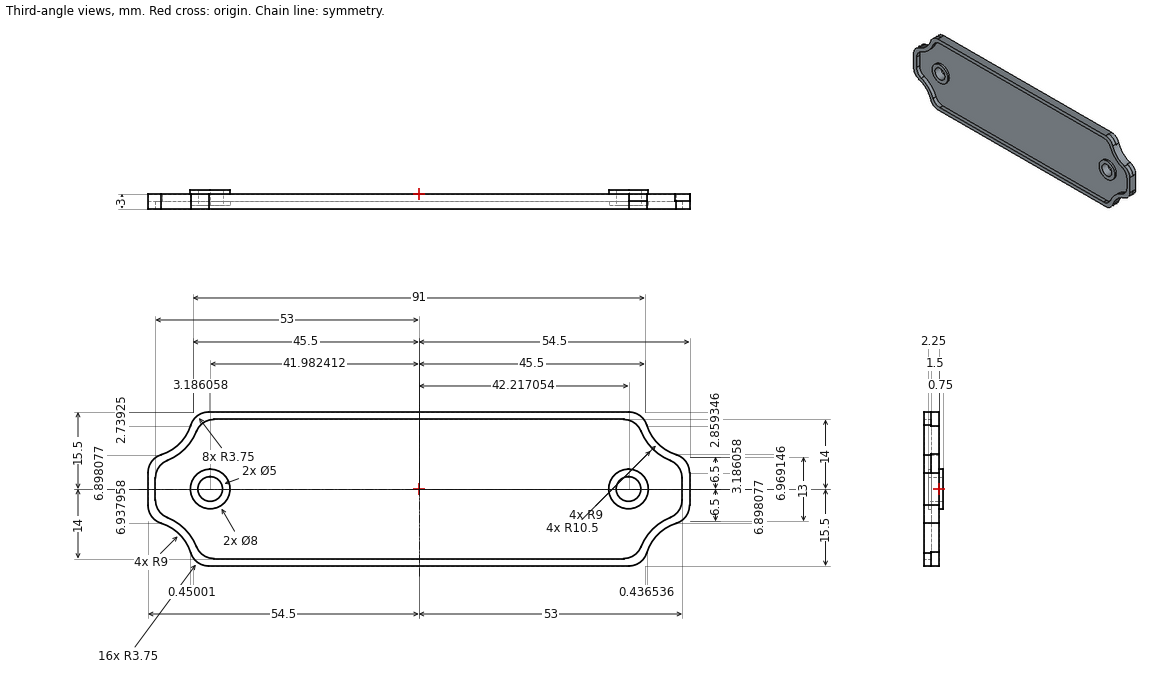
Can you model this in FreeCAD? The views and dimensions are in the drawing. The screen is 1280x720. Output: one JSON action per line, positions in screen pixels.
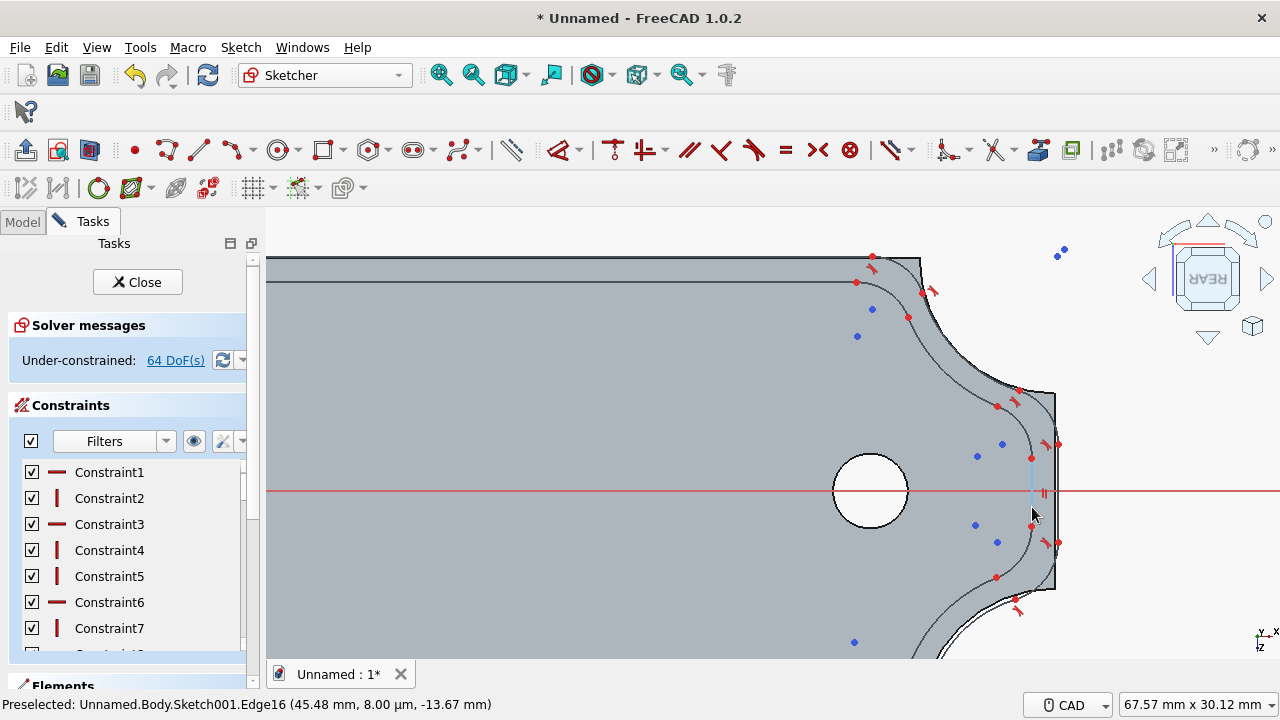
{"action": "left_click", "coordinate": [1032, 506]}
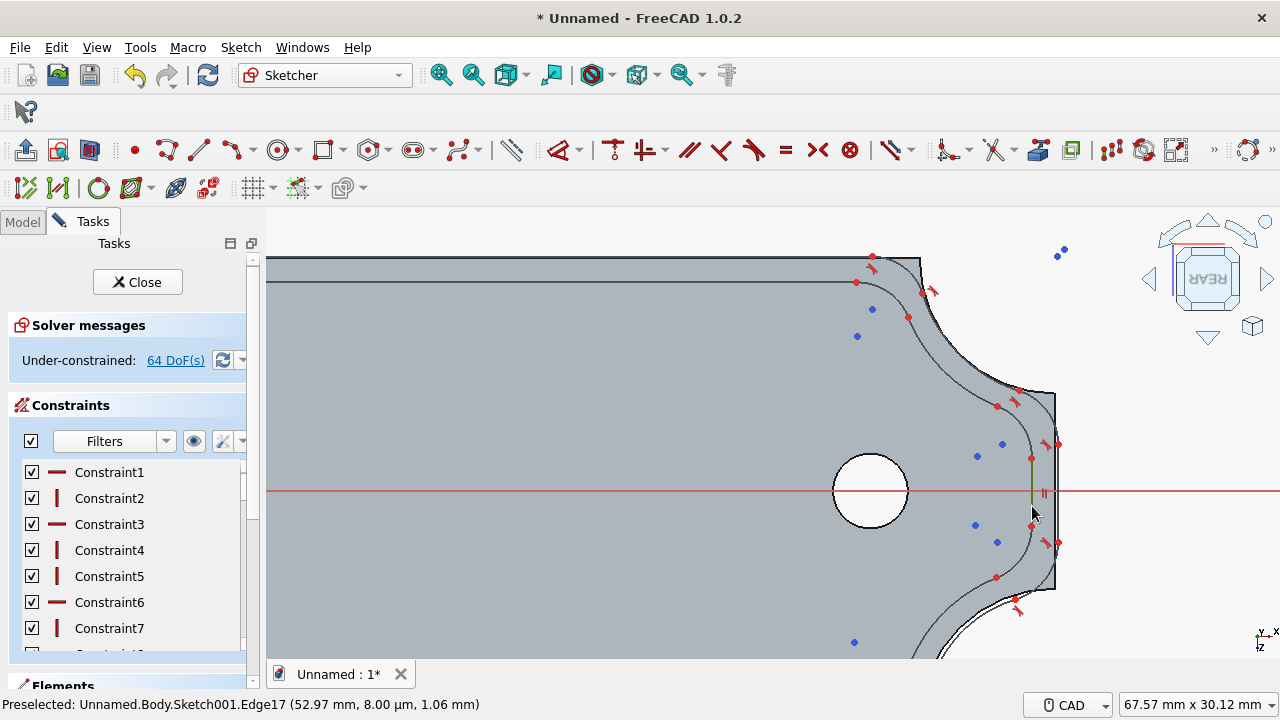
{"action": "left_click", "coordinate": [1013, 567]}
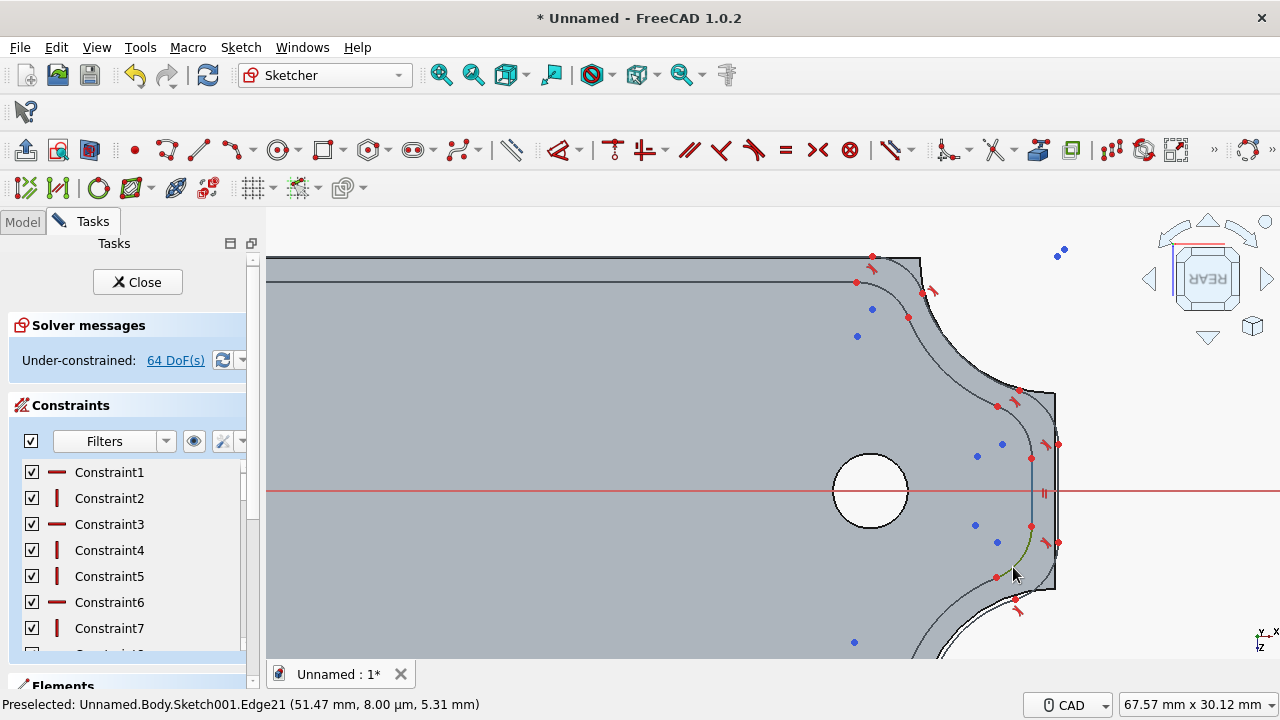
{"action": "left_click", "coordinate": [754, 150]}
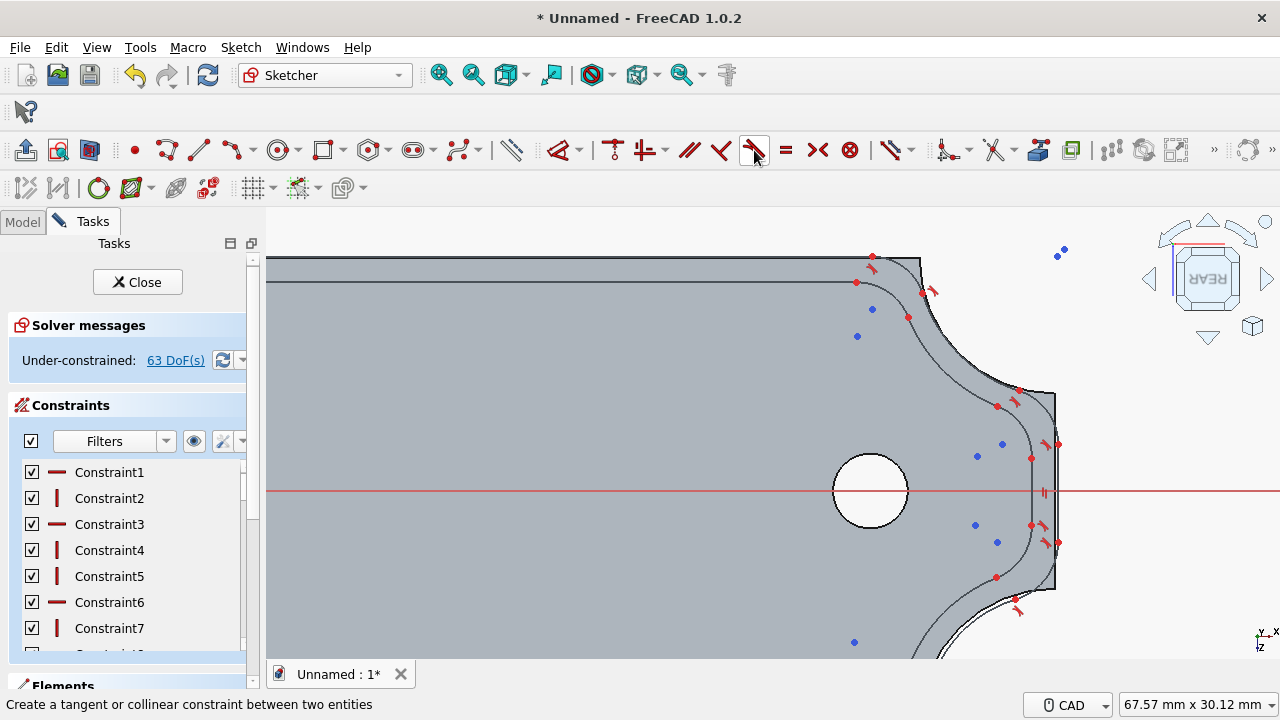
{"action": "left_click", "coordinate": [1032, 478]}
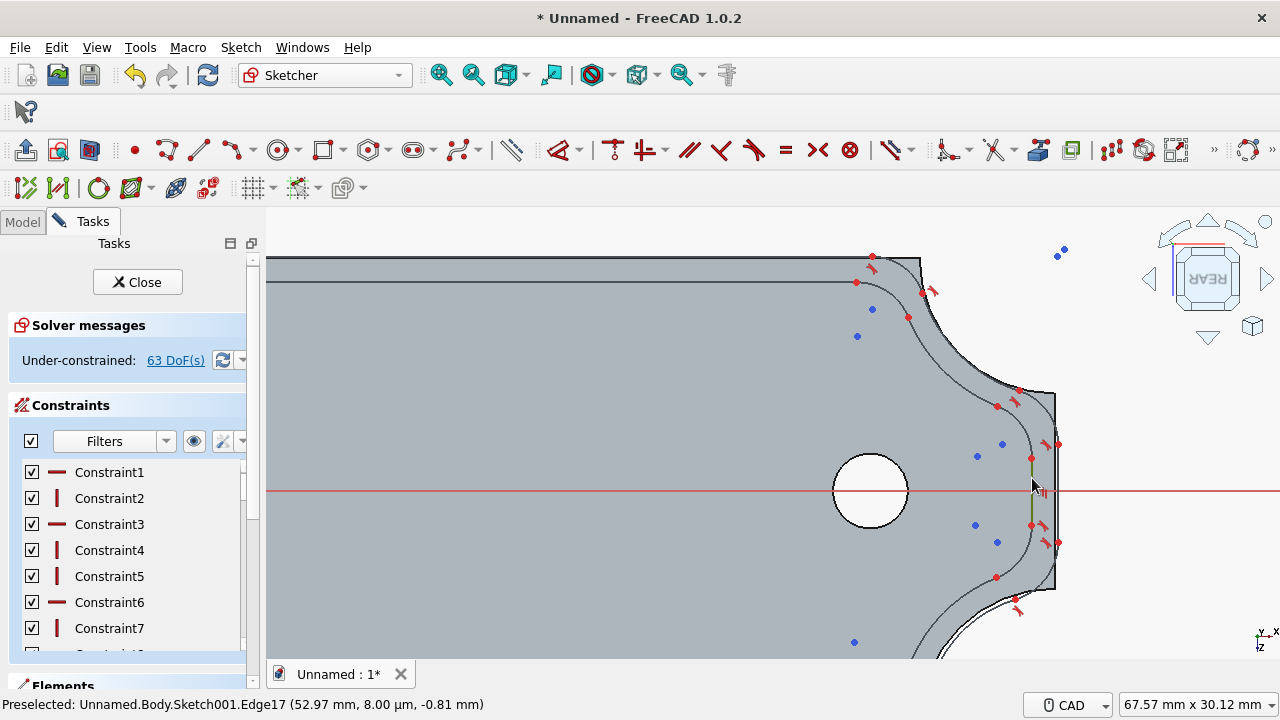
{"action": "left_click", "coordinate": [1029, 439]}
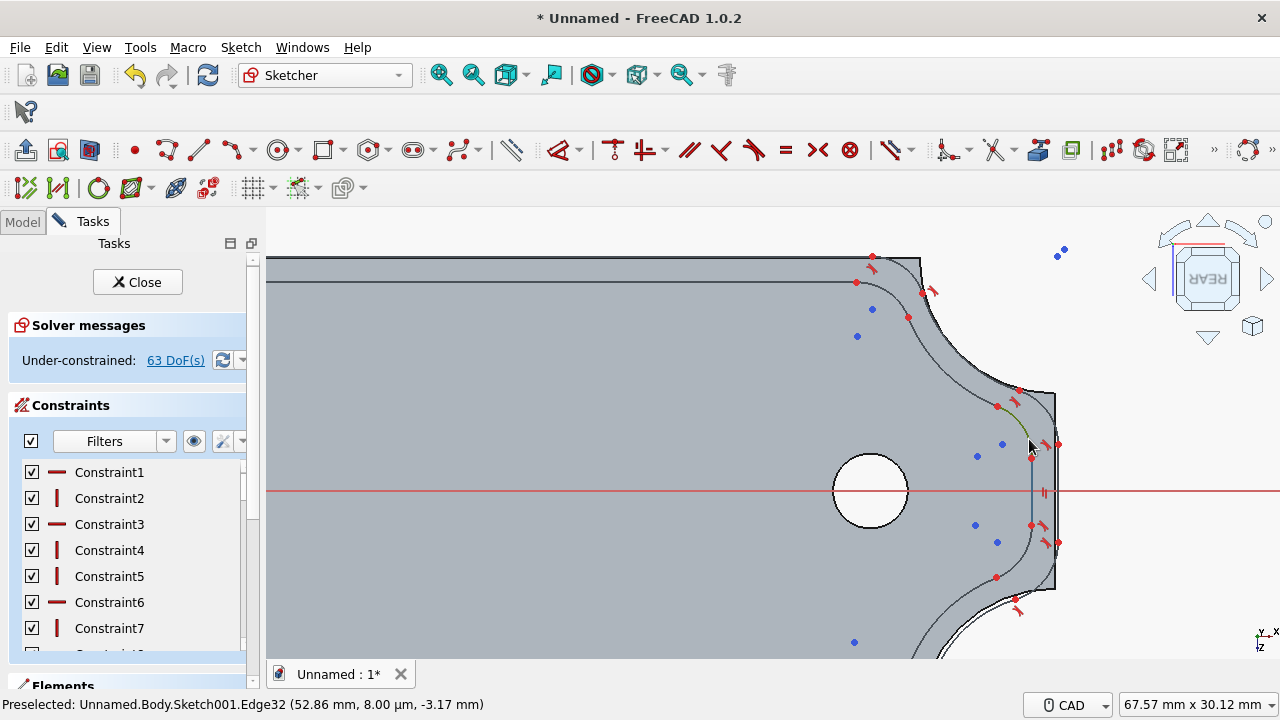
{"action": "left_click", "coordinate": [754, 150]}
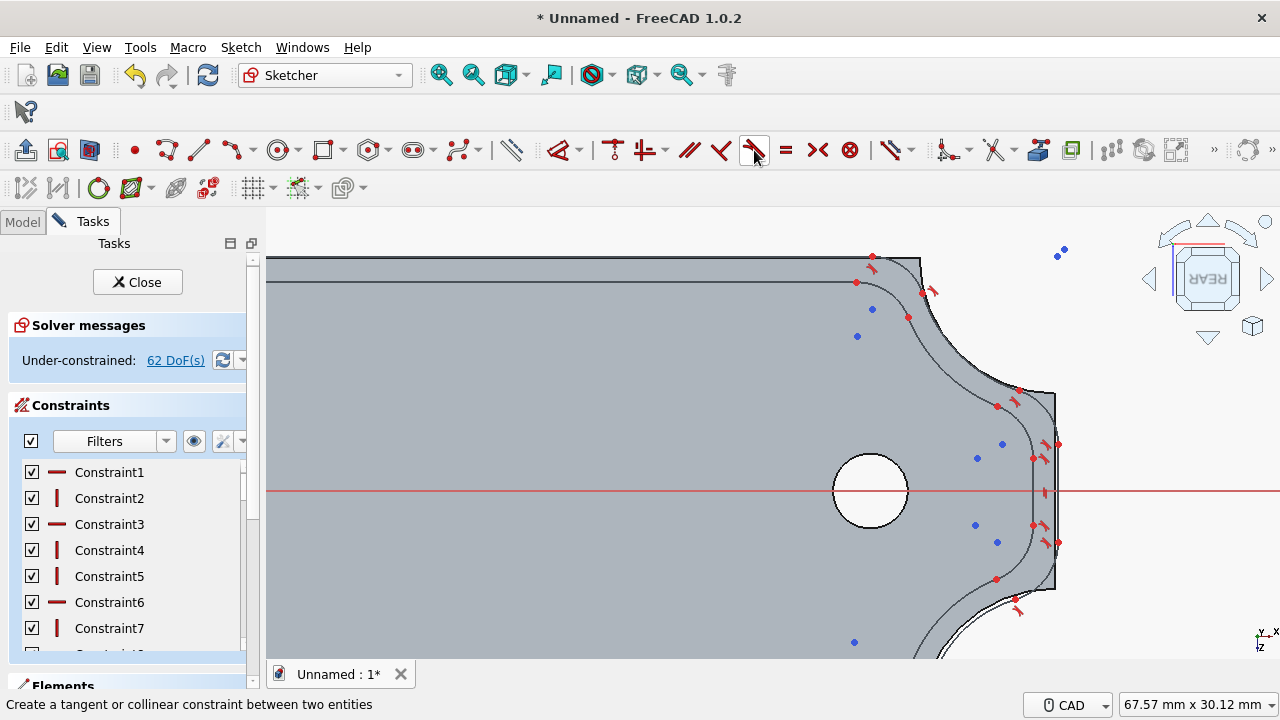
{"action": "scroll", "coordinate": [977, 399], "scroll_direction": "down", "scroll_amount": 5}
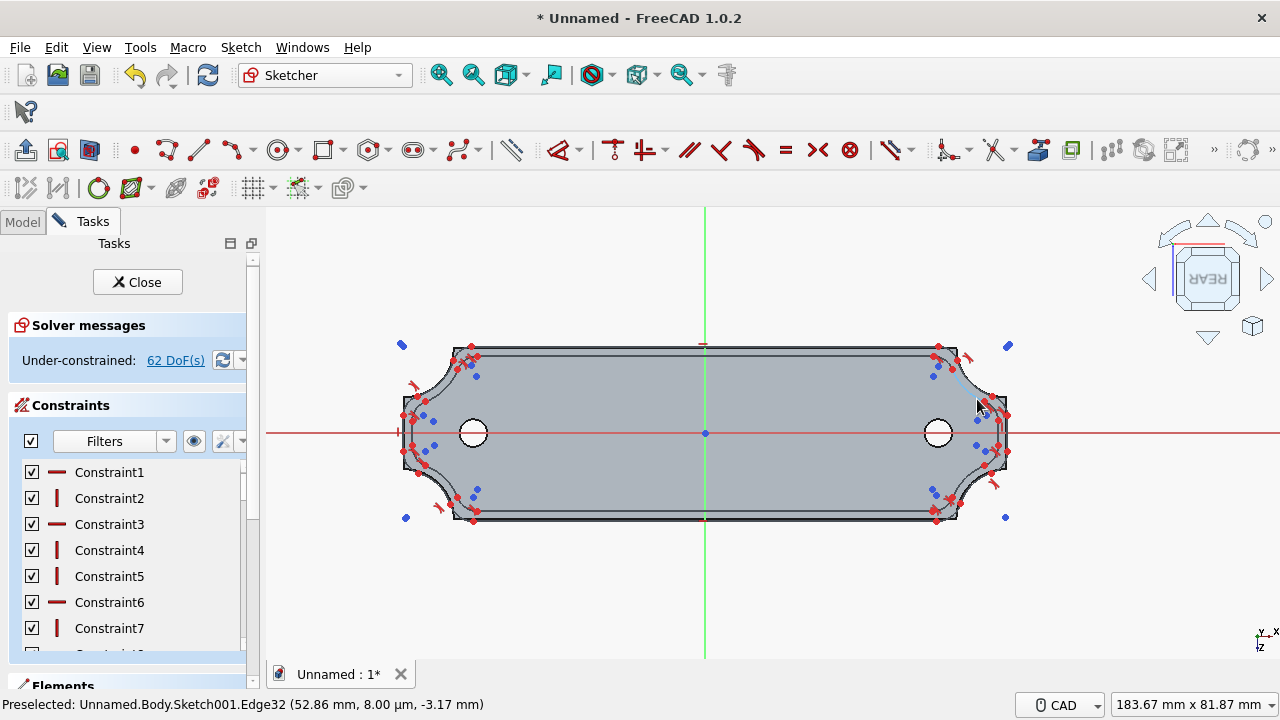
{"action": "scroll", "coordinate": [796, 511], "scroll_direction": "up", "scroll_amount": 2}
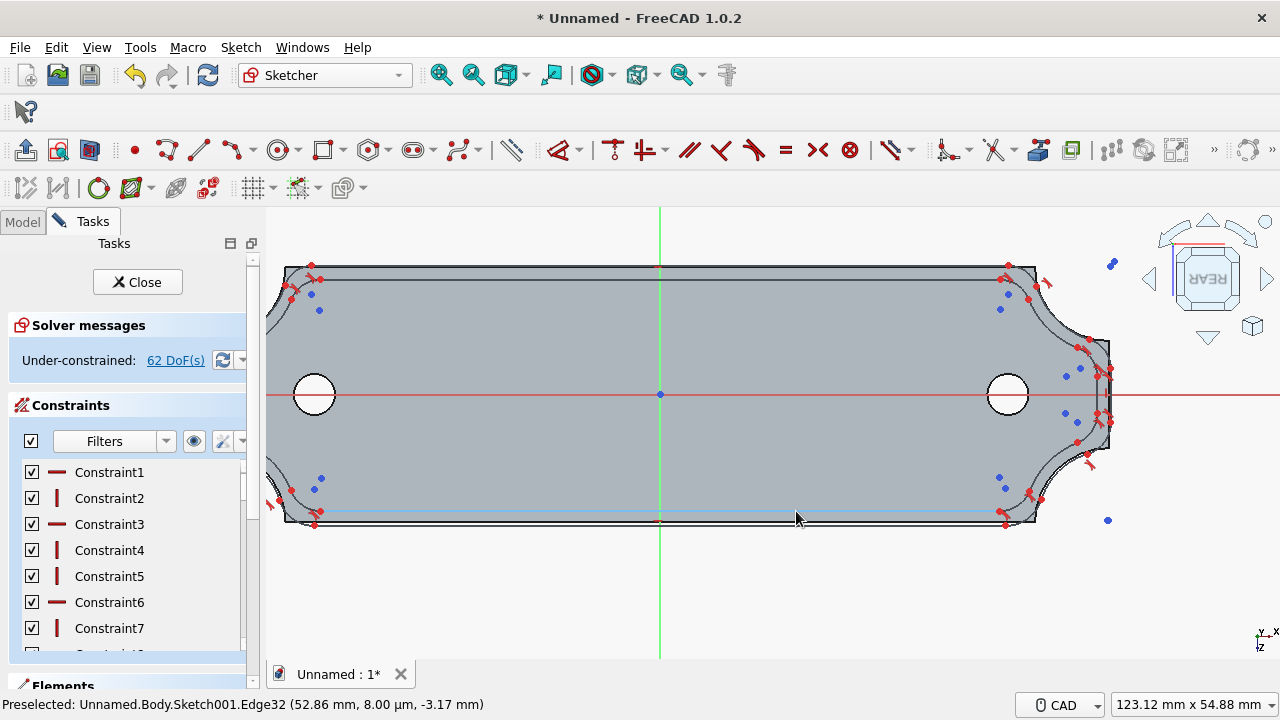
{"action": "left_click", "coordinate": [796, 511]}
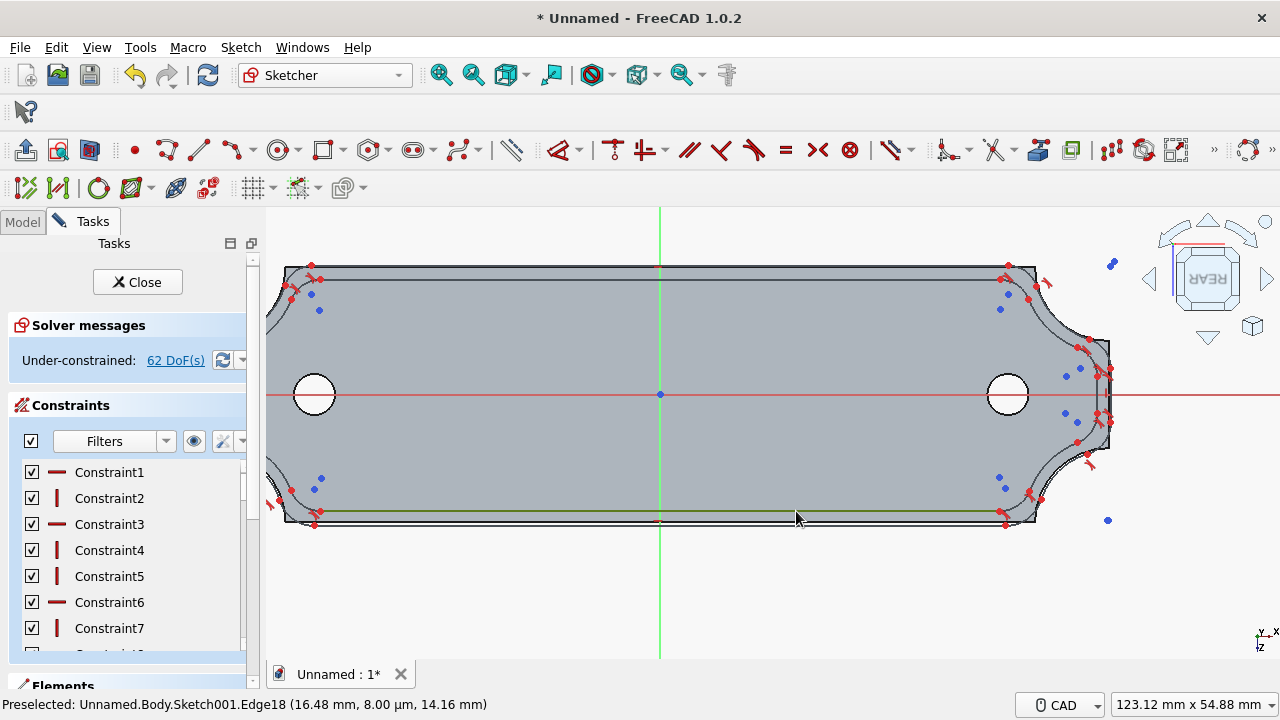
{"action": "left_click", "coordinate": [1024, 501]}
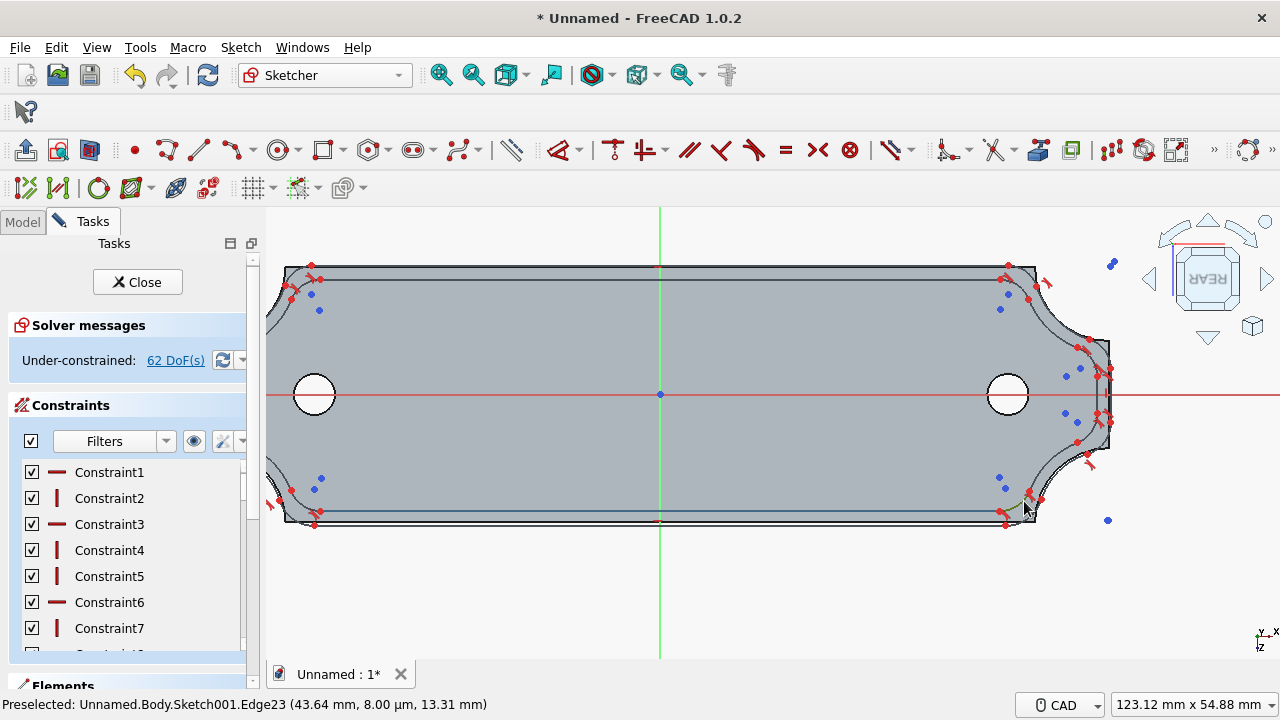
{"action": "left_click", "coordinate": [754, 150]}